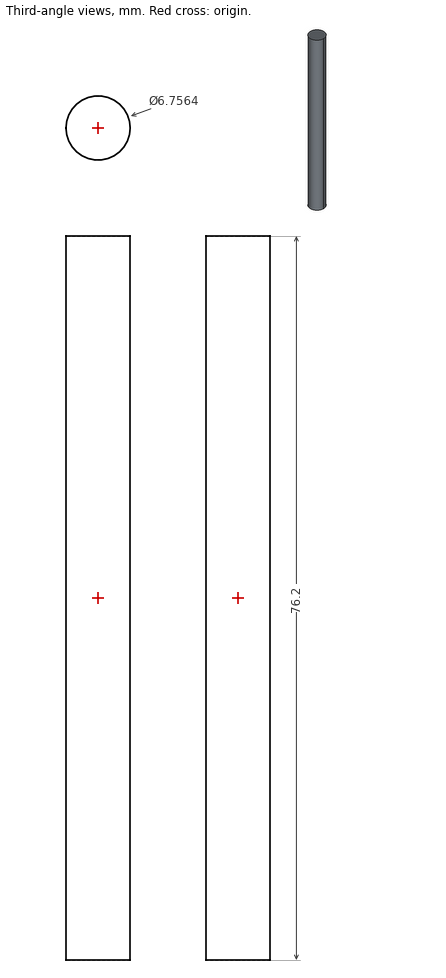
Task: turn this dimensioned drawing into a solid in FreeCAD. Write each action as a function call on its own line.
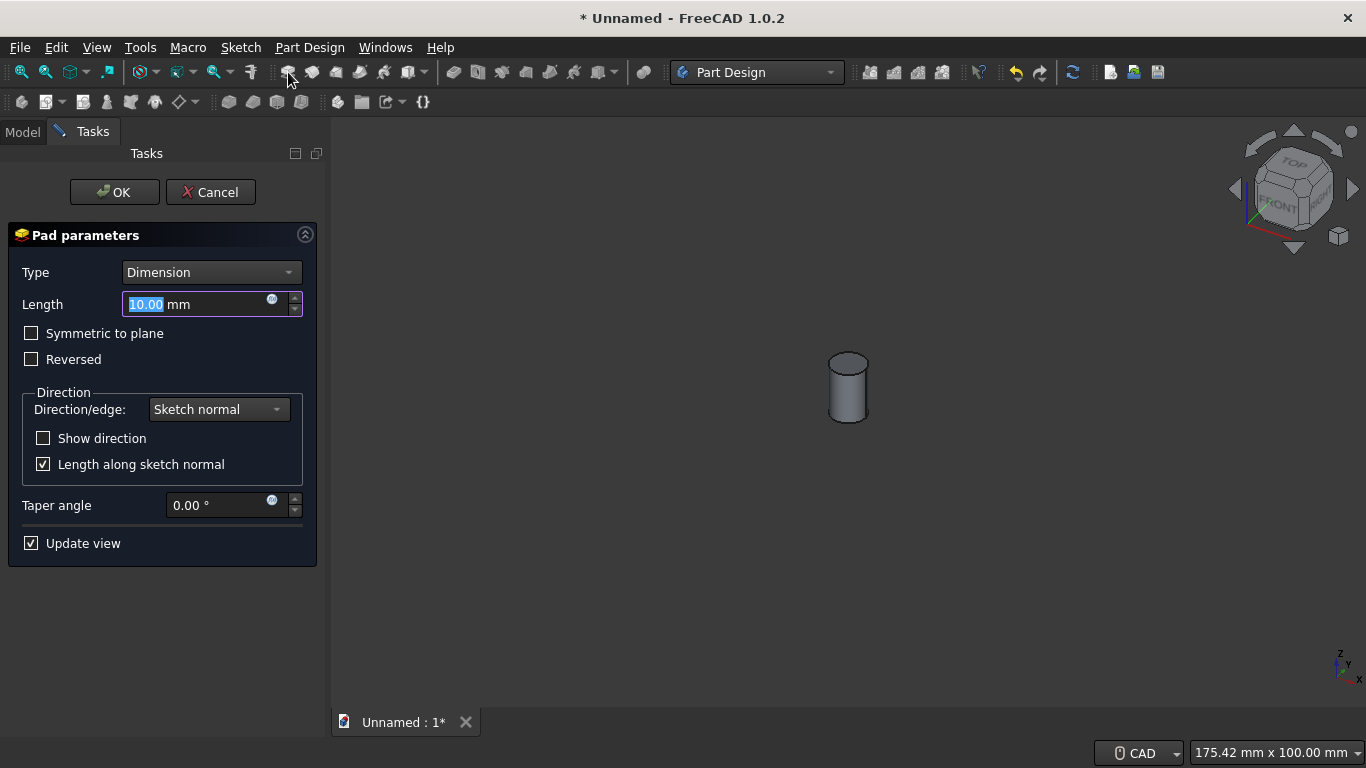
text(76.2)
key(Tab)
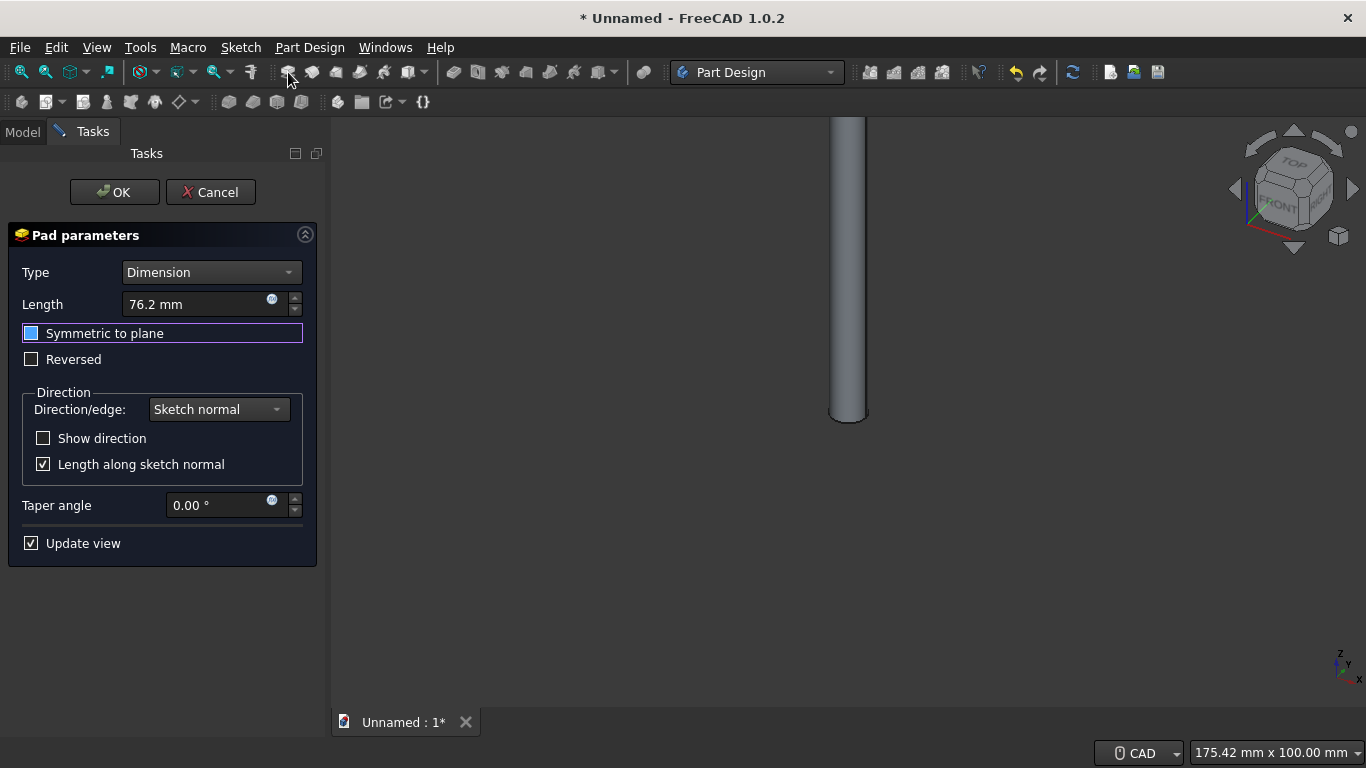
click(30, 333)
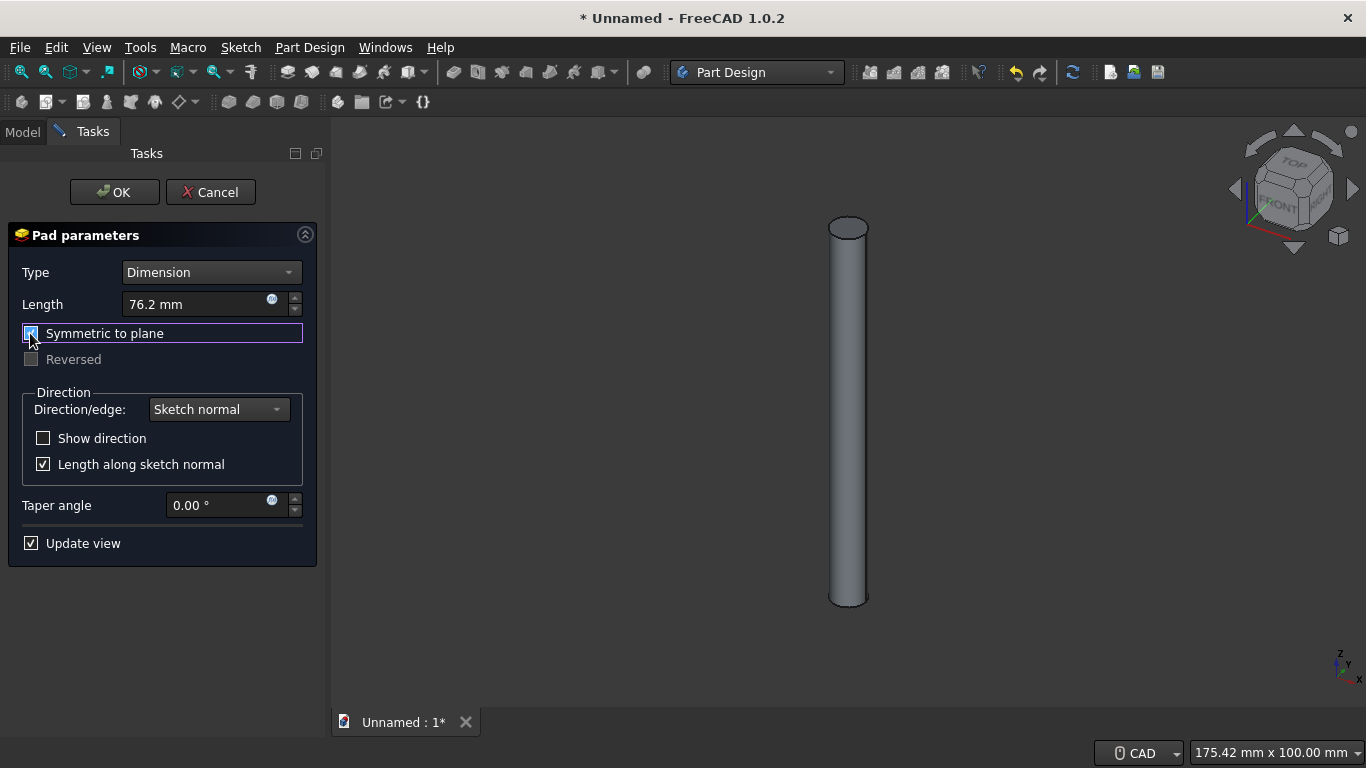
click(115, 192)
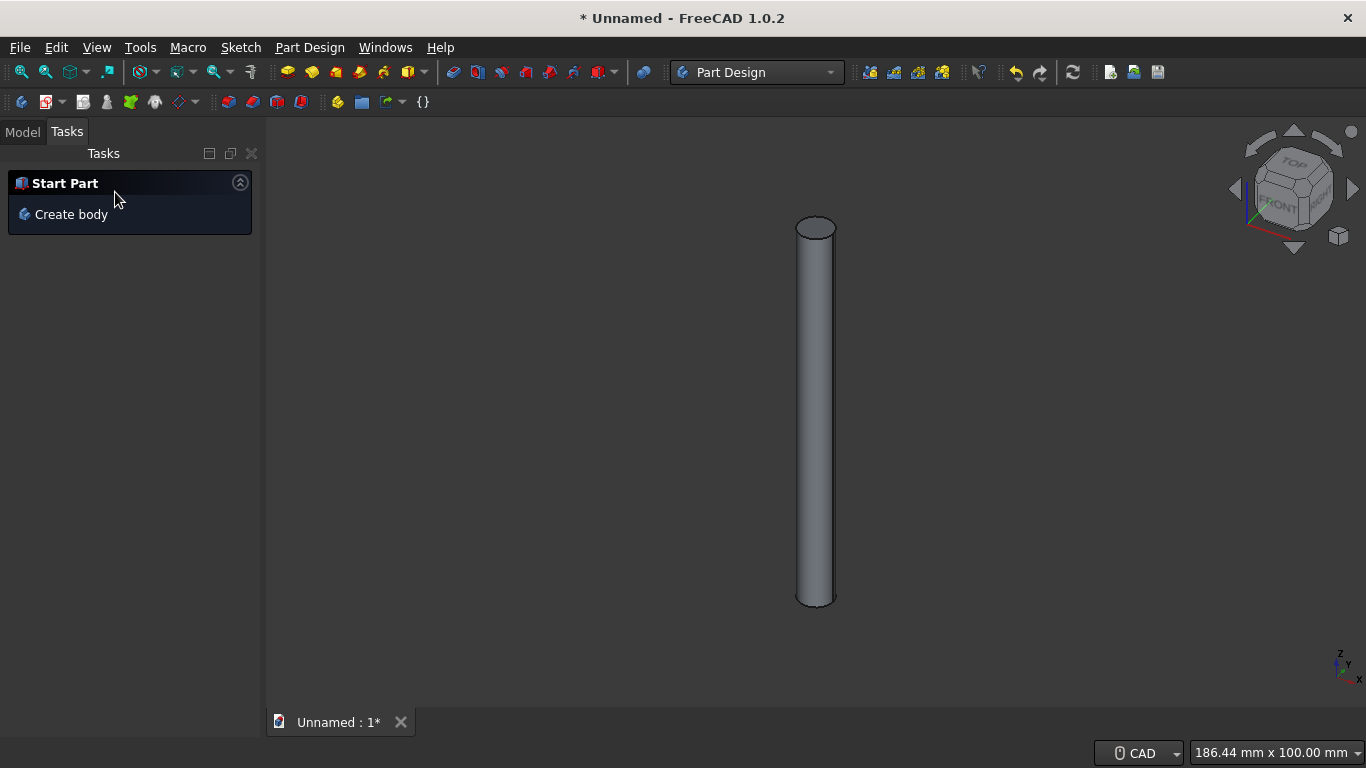
key(0)